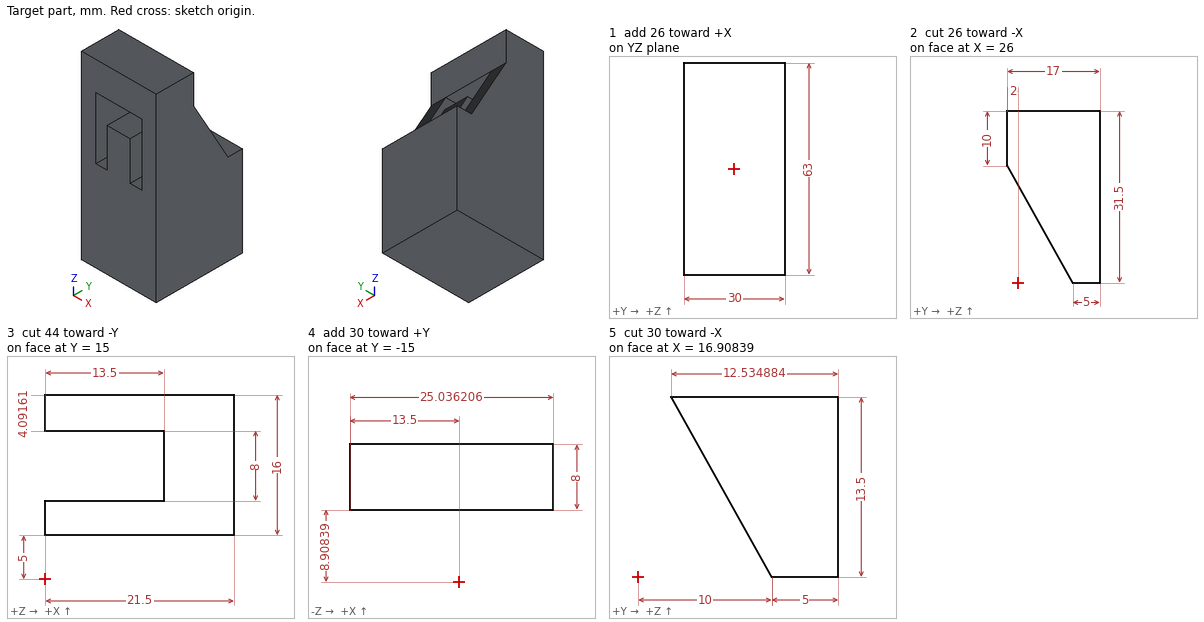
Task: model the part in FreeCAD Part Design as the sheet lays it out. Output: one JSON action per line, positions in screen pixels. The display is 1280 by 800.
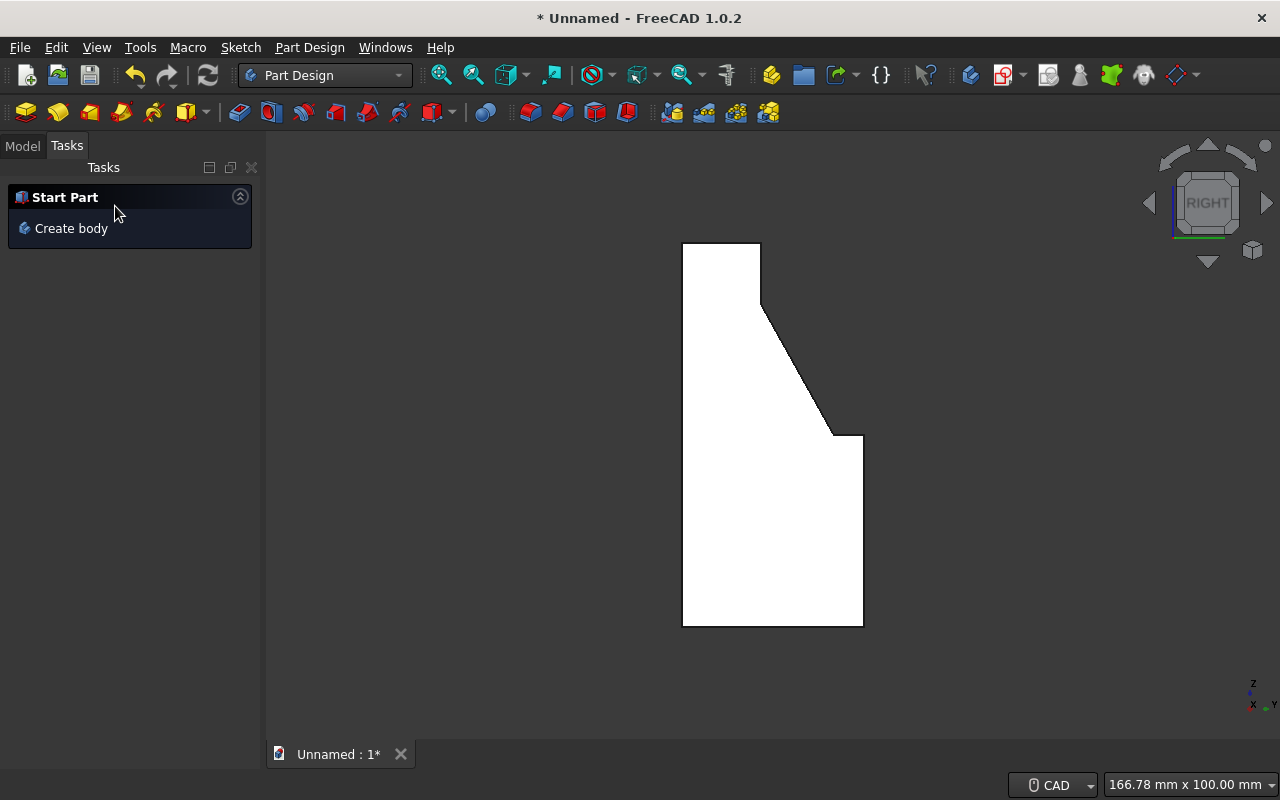
{"action": "key", "text": "0"}